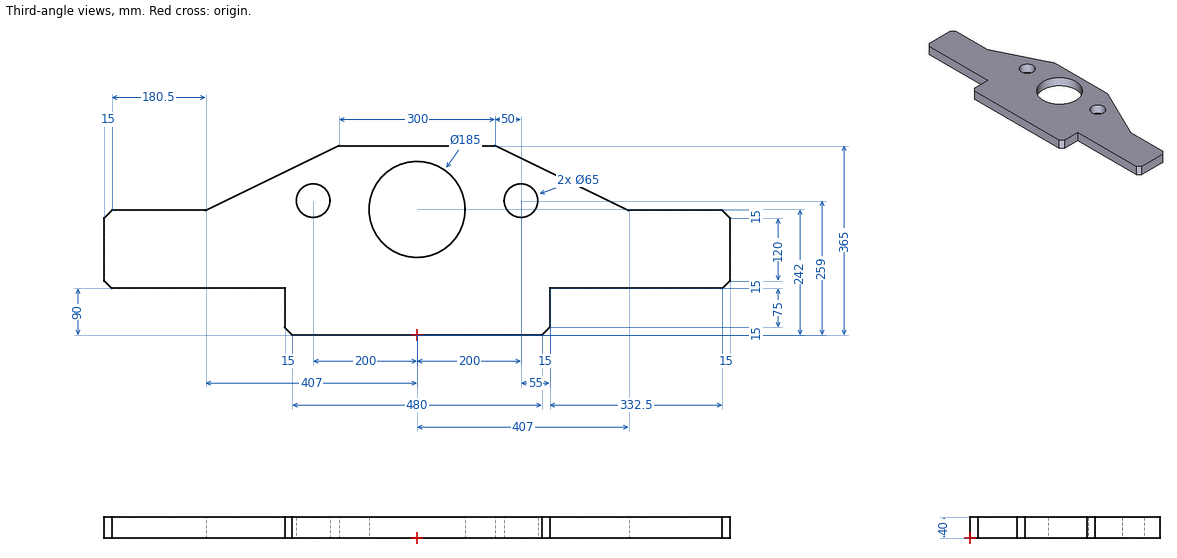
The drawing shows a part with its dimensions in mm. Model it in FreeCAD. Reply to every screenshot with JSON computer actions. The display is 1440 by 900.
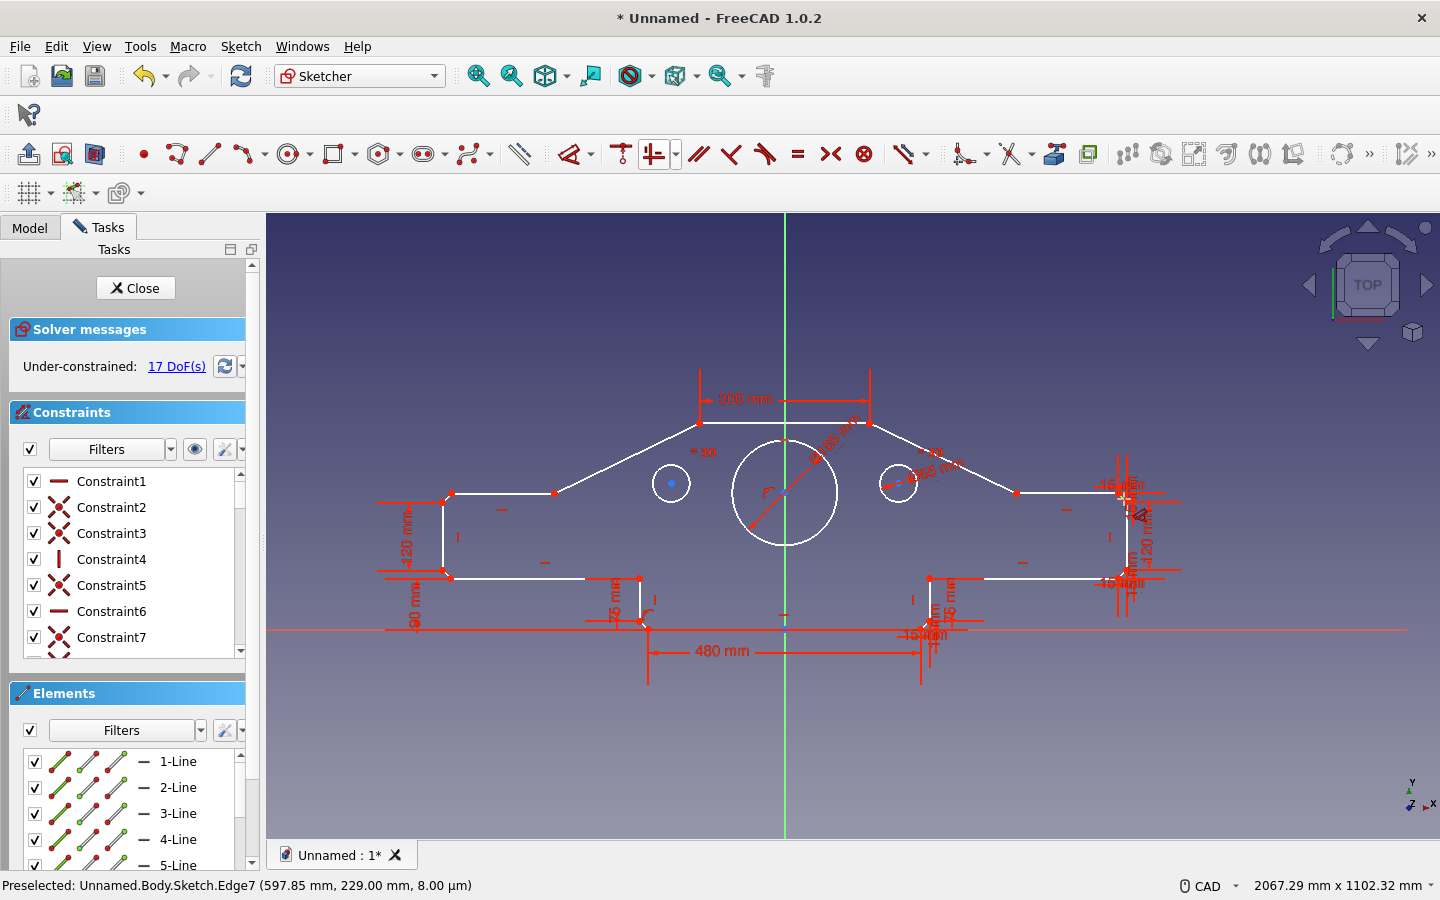
{"action": "scroll", "coordinate": [449, 497], "scroll_direction": "up", "scroll_amount": 8}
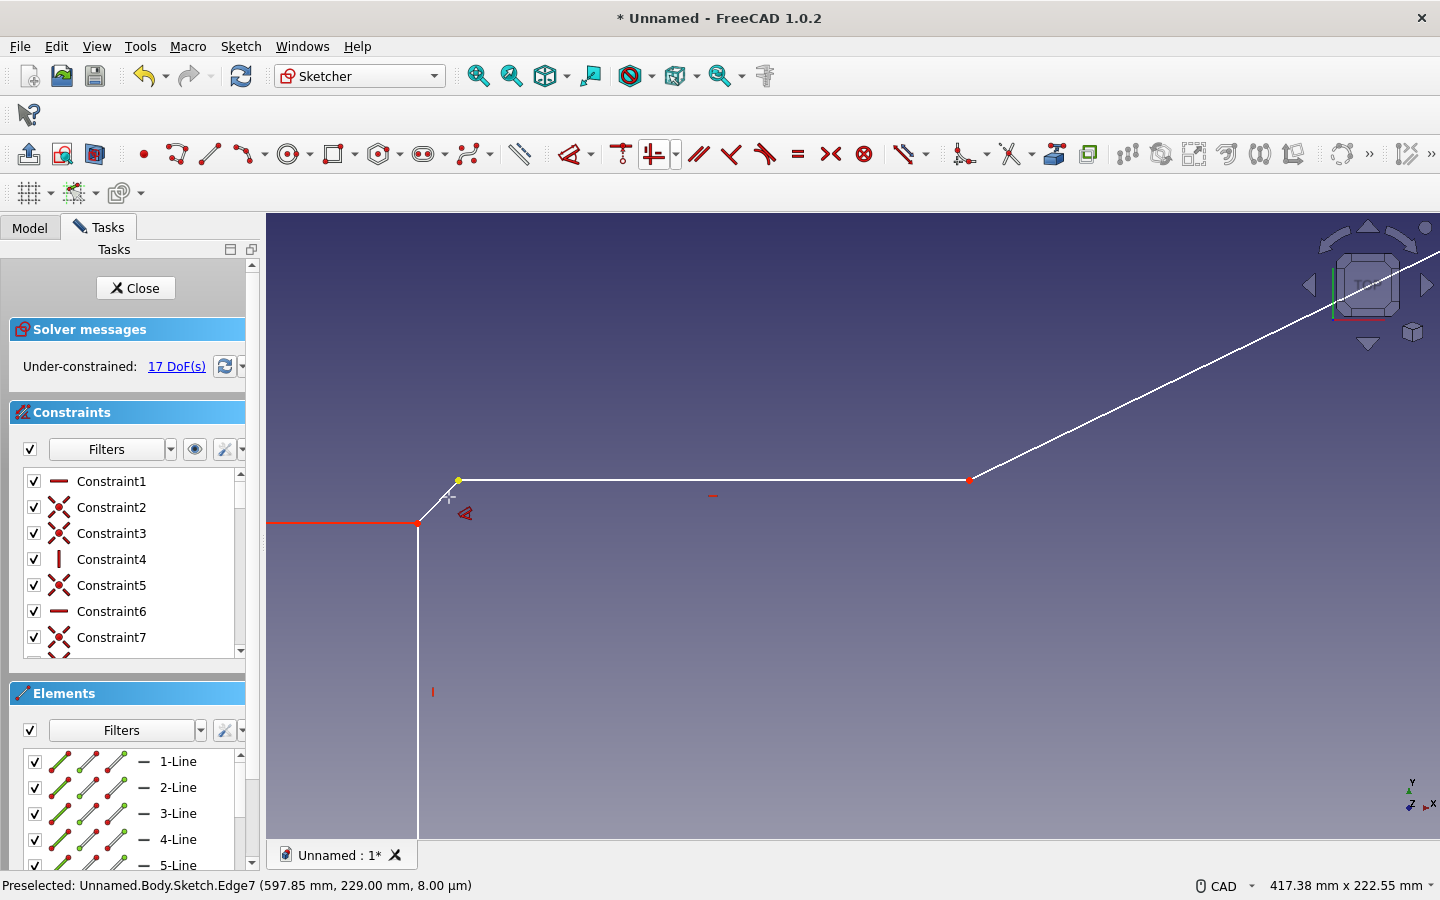
{"action": "left_click", "coordinate": [447, 493]}
{"action": "left_click", "coordinate": [438, 446]}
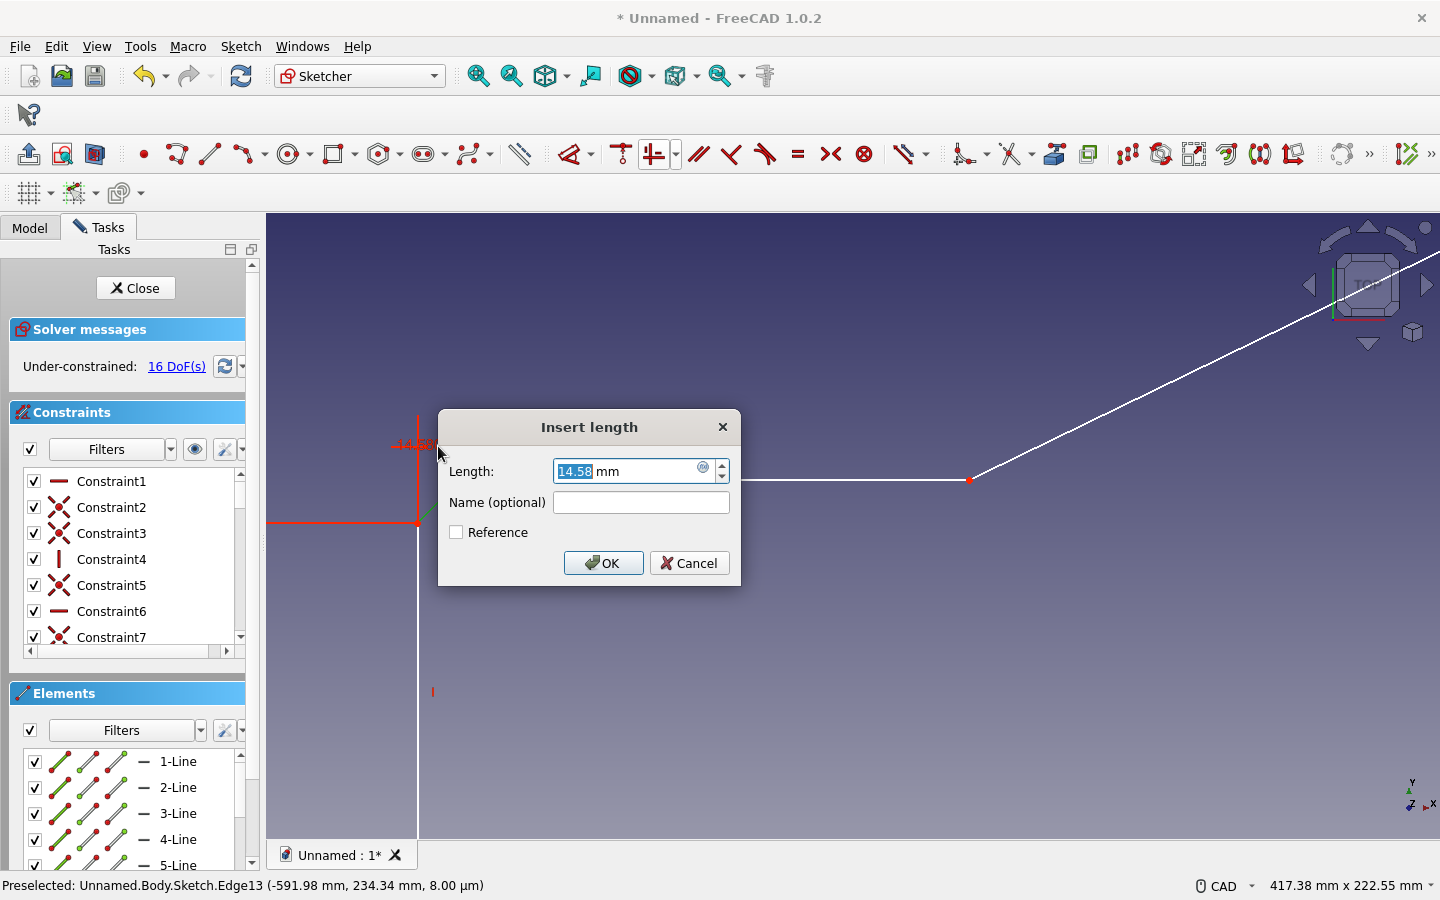
{"action": "type", "text": "15"}
{"action": "key", "text": "Return"}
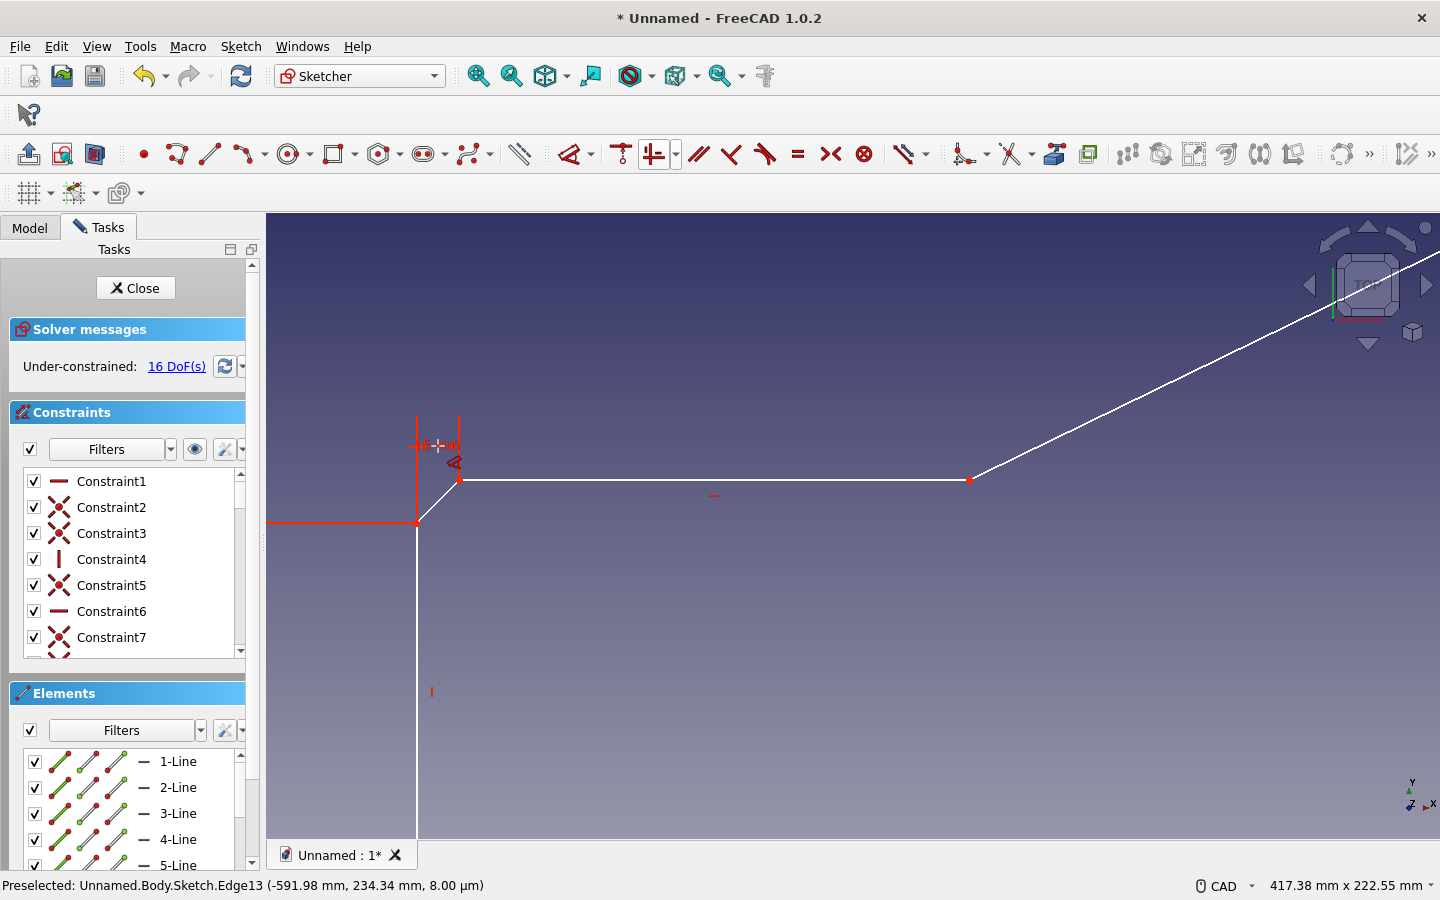
{"action": "left_click", "coordinate": [446, 493]}
{"action": "left_click", "coordinate": [383, 502]}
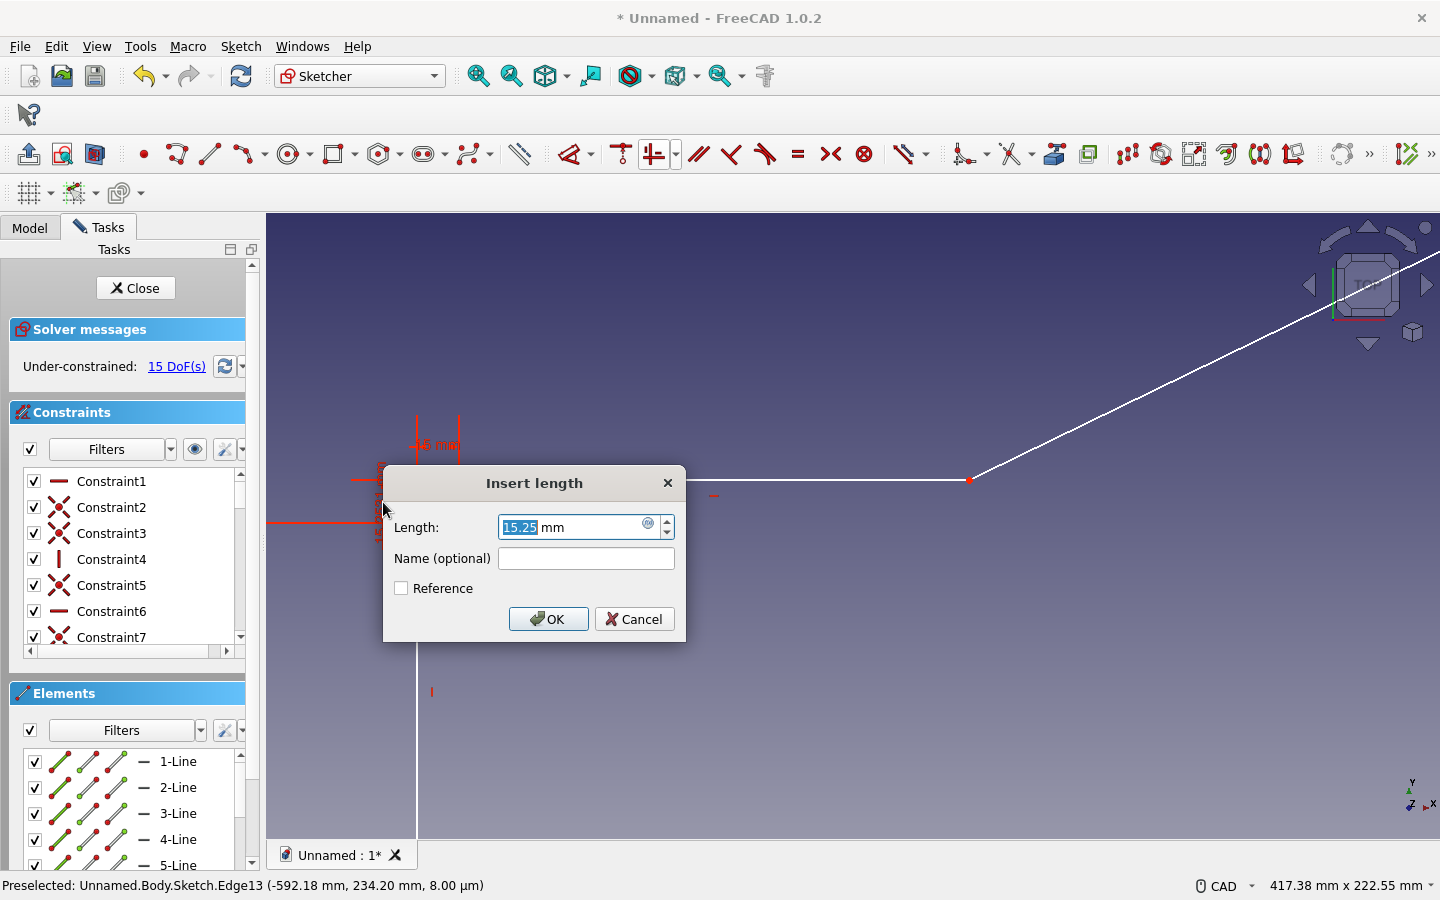
{"action": "type", "text": "15"}
{"action": "key", "text": "Return"}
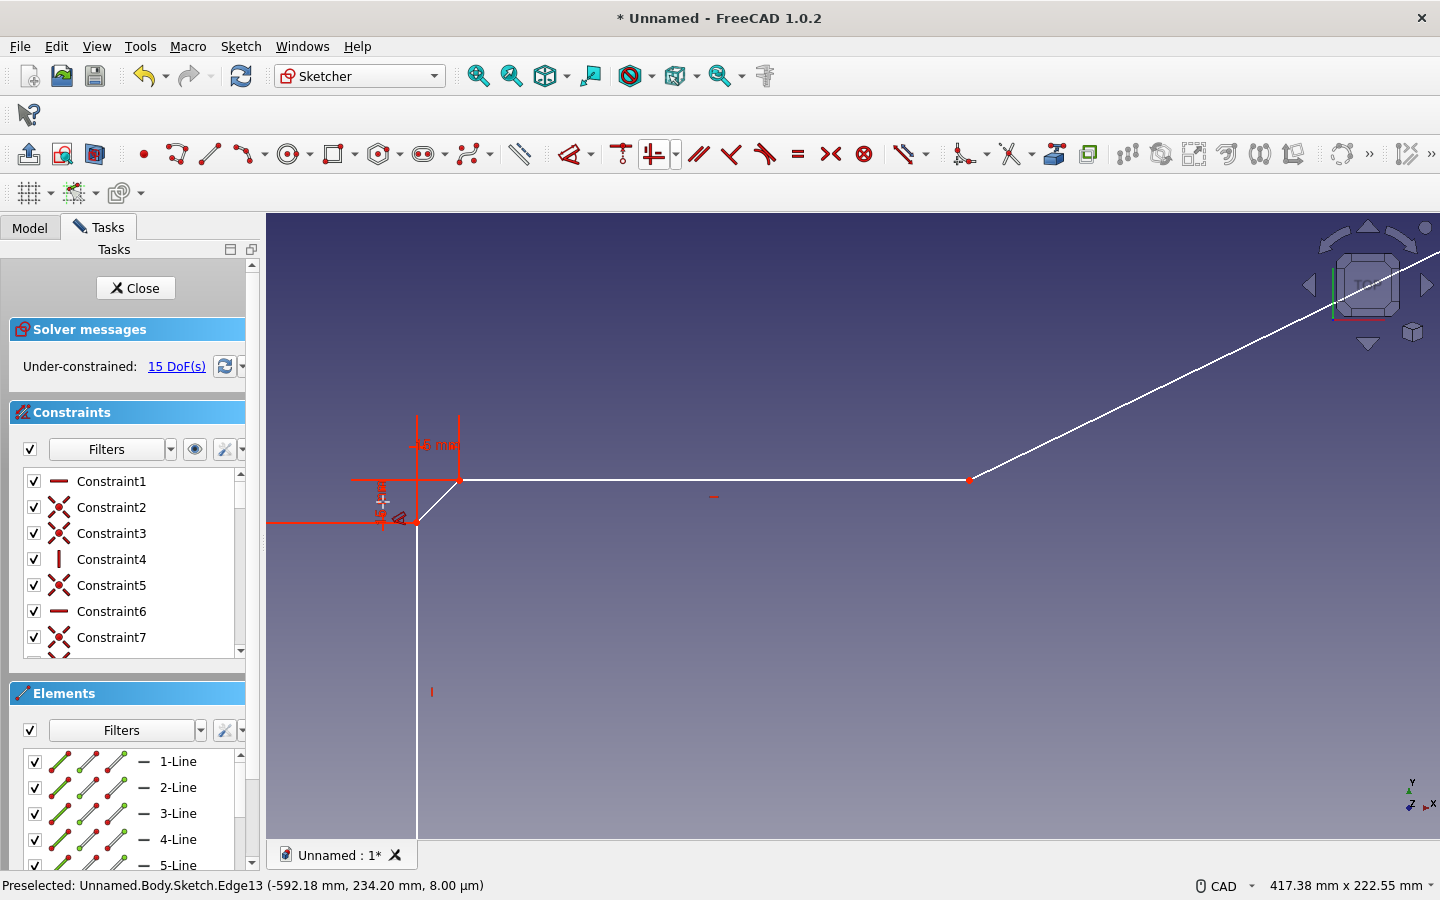
{"action": "scroll", "coordinate": [449, 497], "scroll_direction": "down", "scroll_amount": 8}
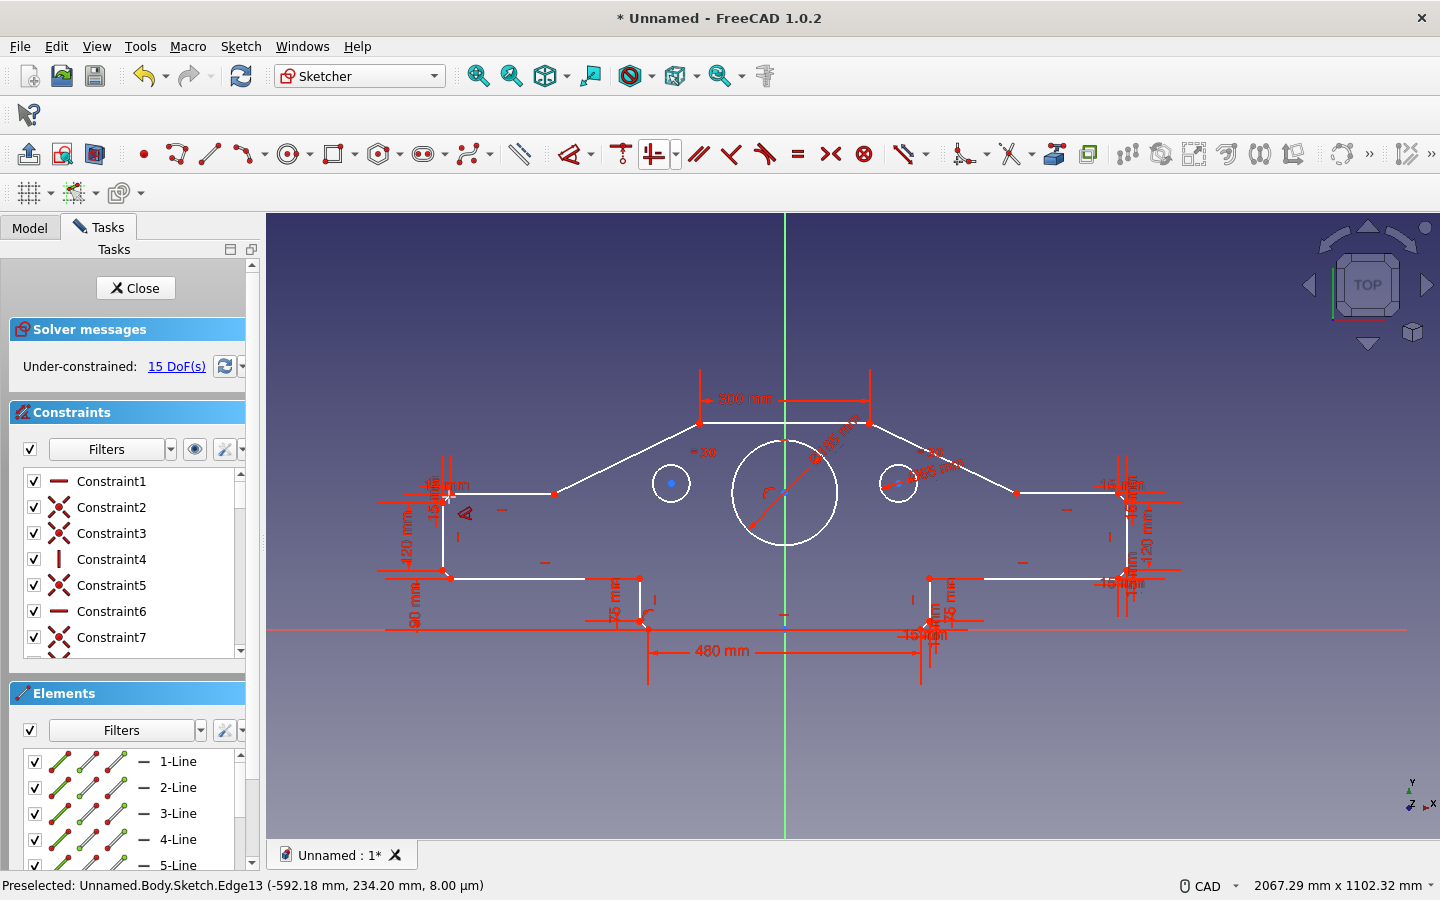
{"action": "scroll", "coordinate": [445, 573], "scroll_direction": "up", "scroll_amount": 8}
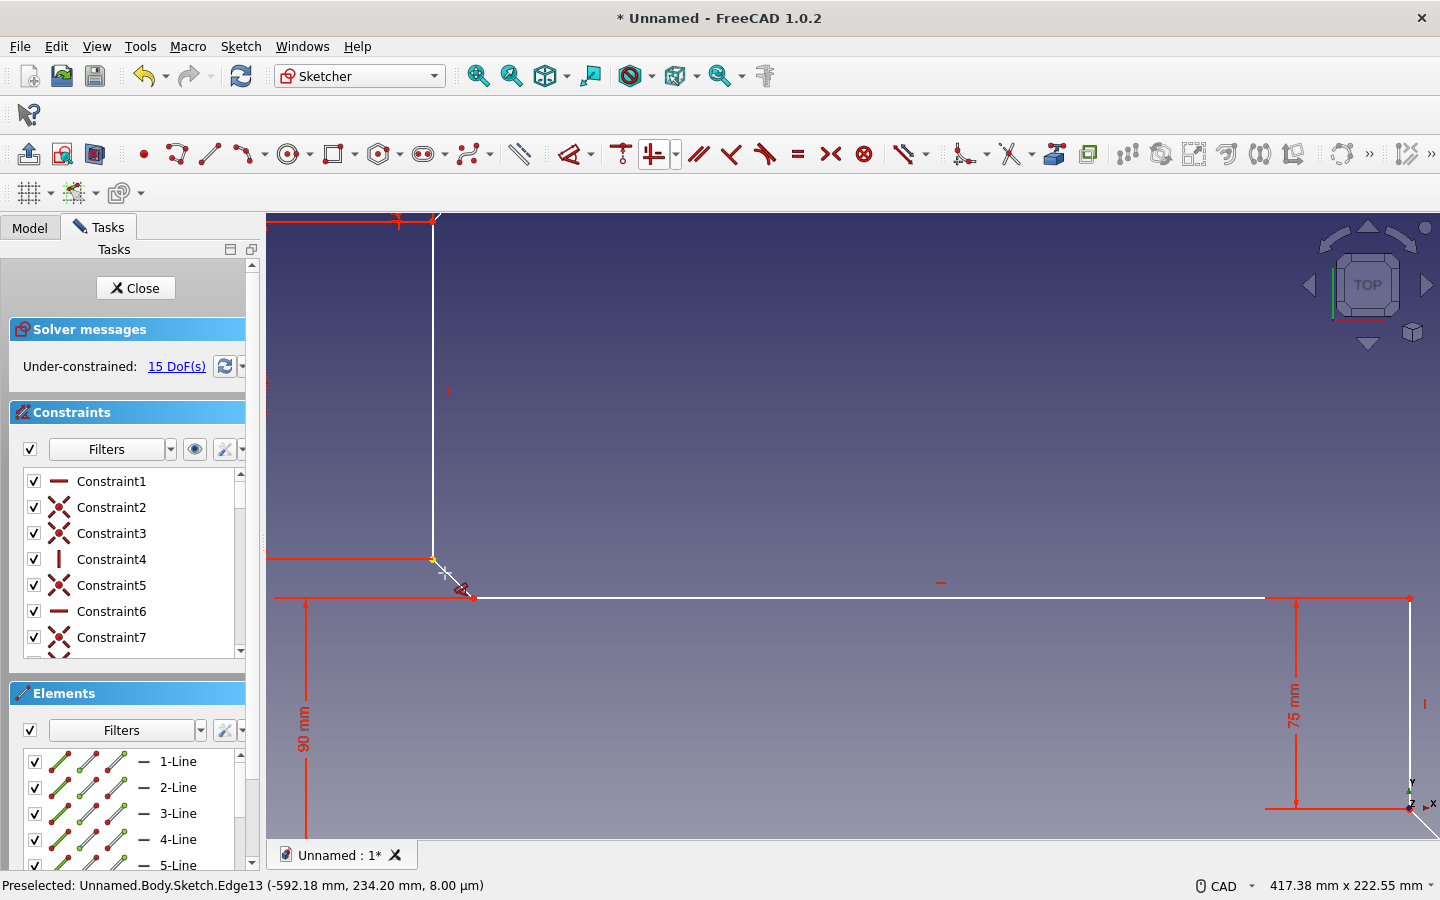
{"action": "left_click", "coordinate": [445, 571]}
{"action": "left_click", "coordinate": [453, 632]}